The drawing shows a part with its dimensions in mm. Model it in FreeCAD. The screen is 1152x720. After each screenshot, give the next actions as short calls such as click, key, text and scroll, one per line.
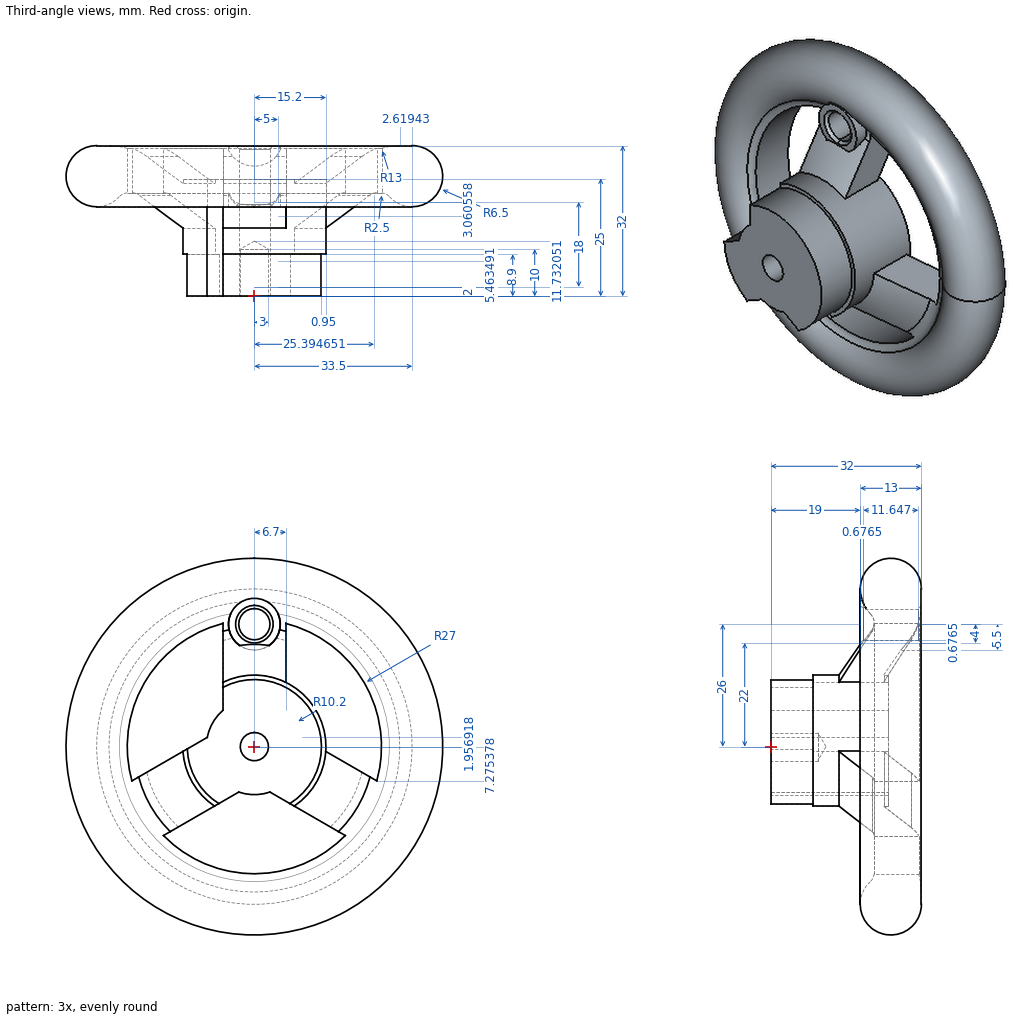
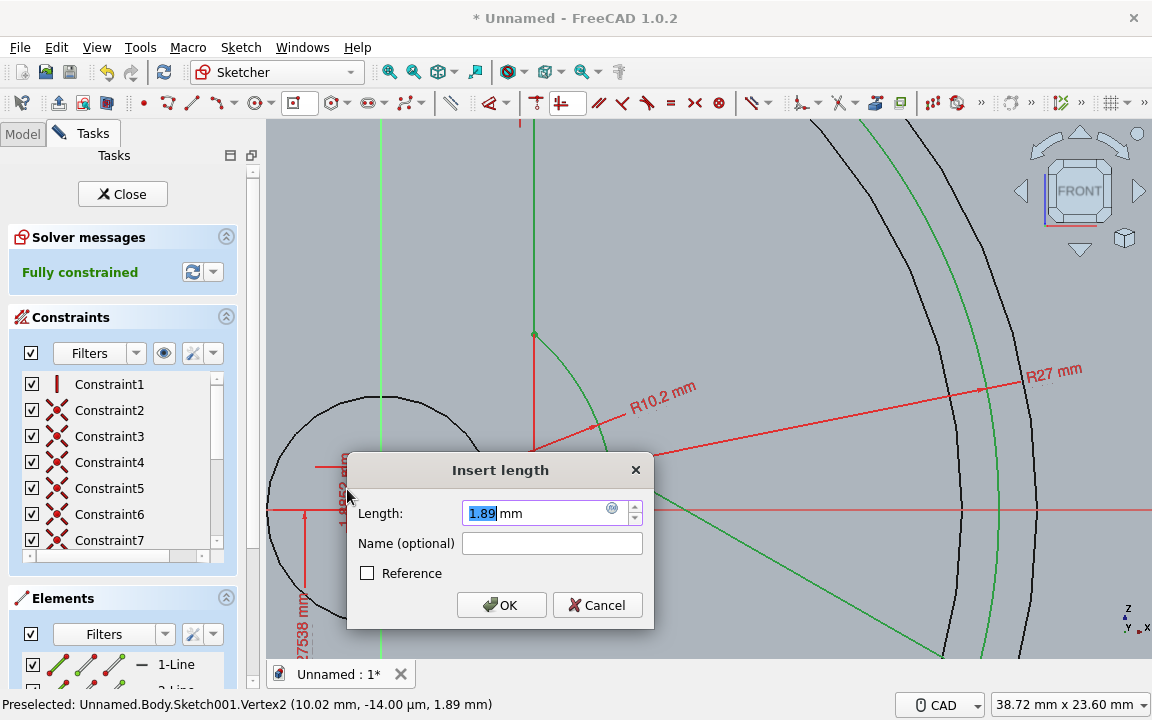
text(1.956918)
key(Return)
key(Escape)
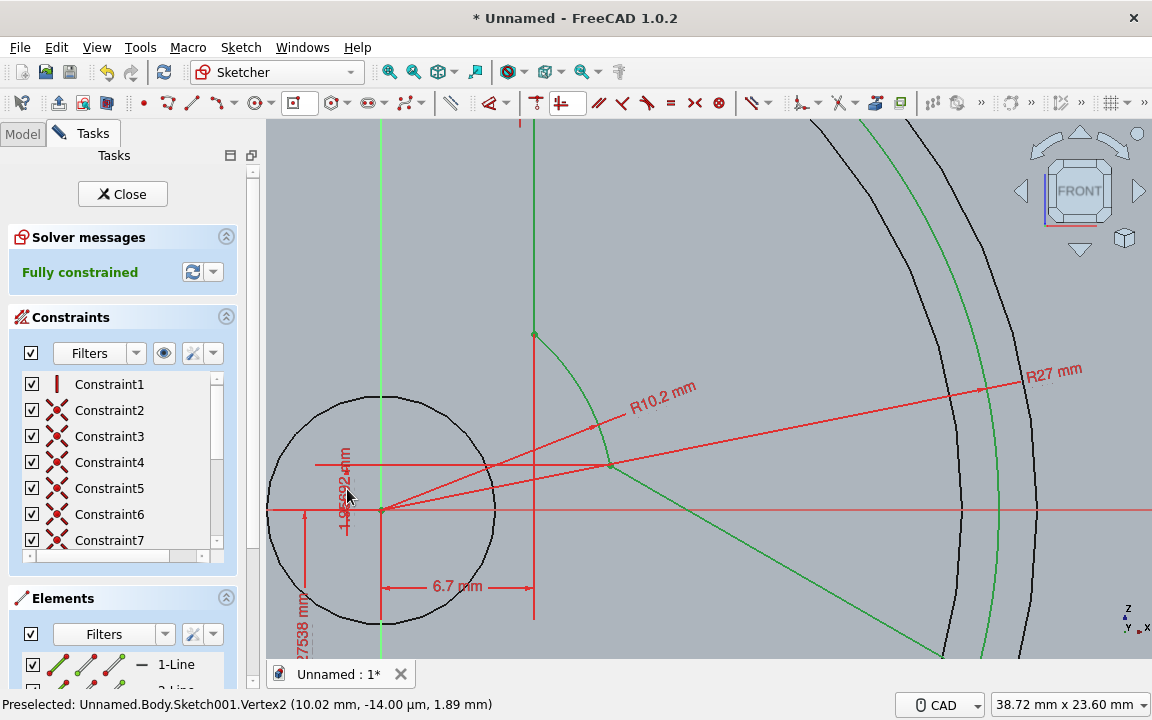
click(123, 194)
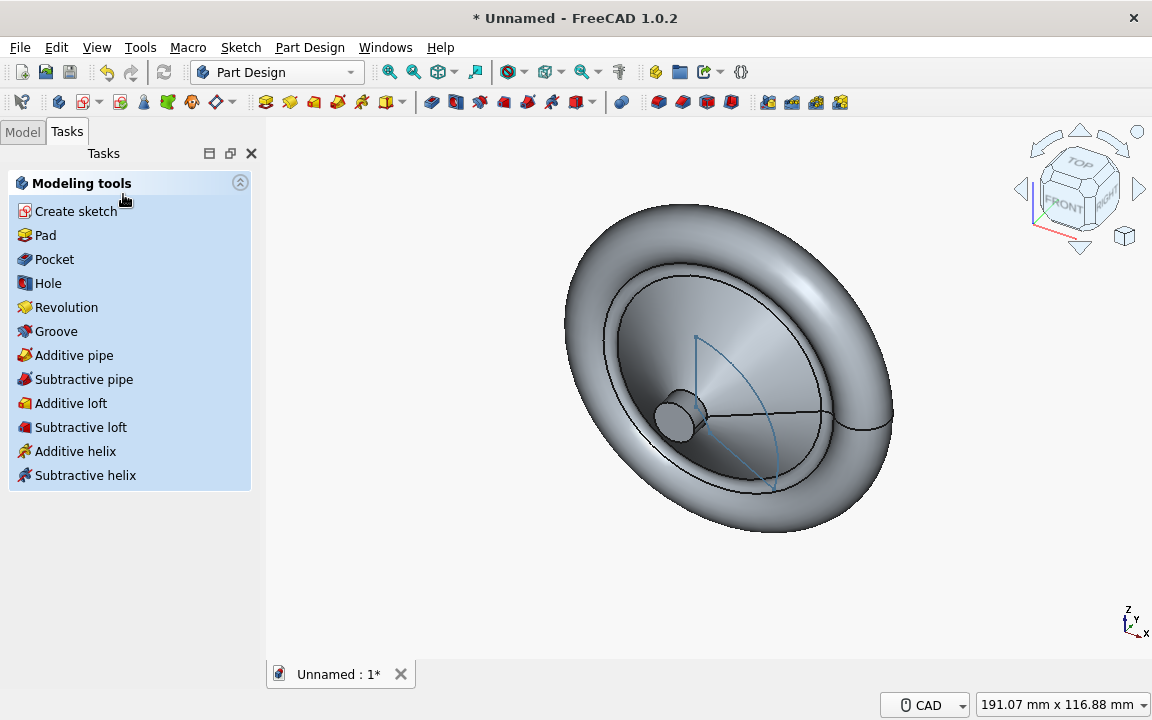
click(432, 102)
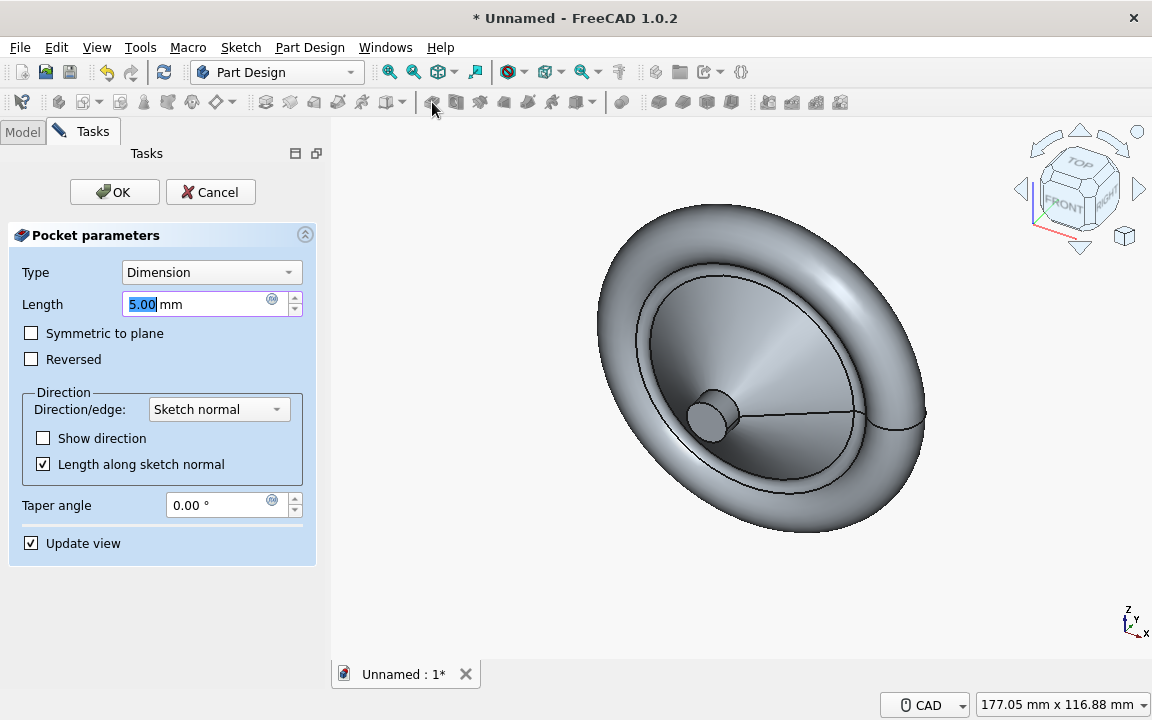
text(32)
key(Tab)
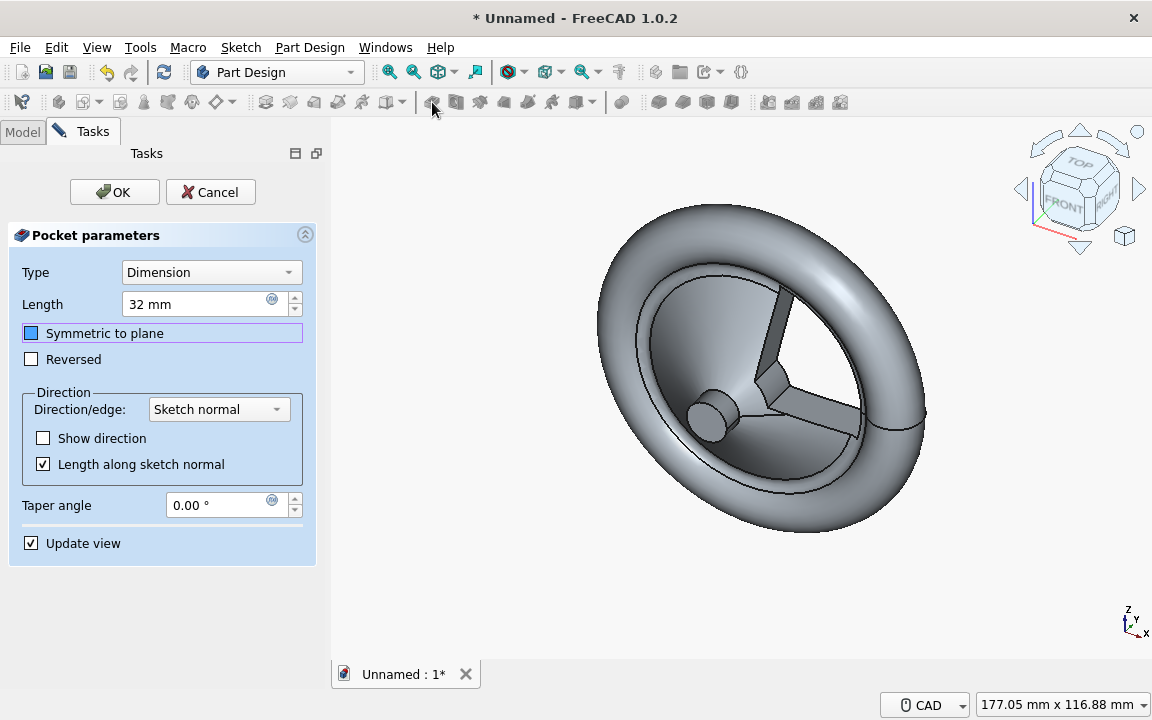
click(115, 192)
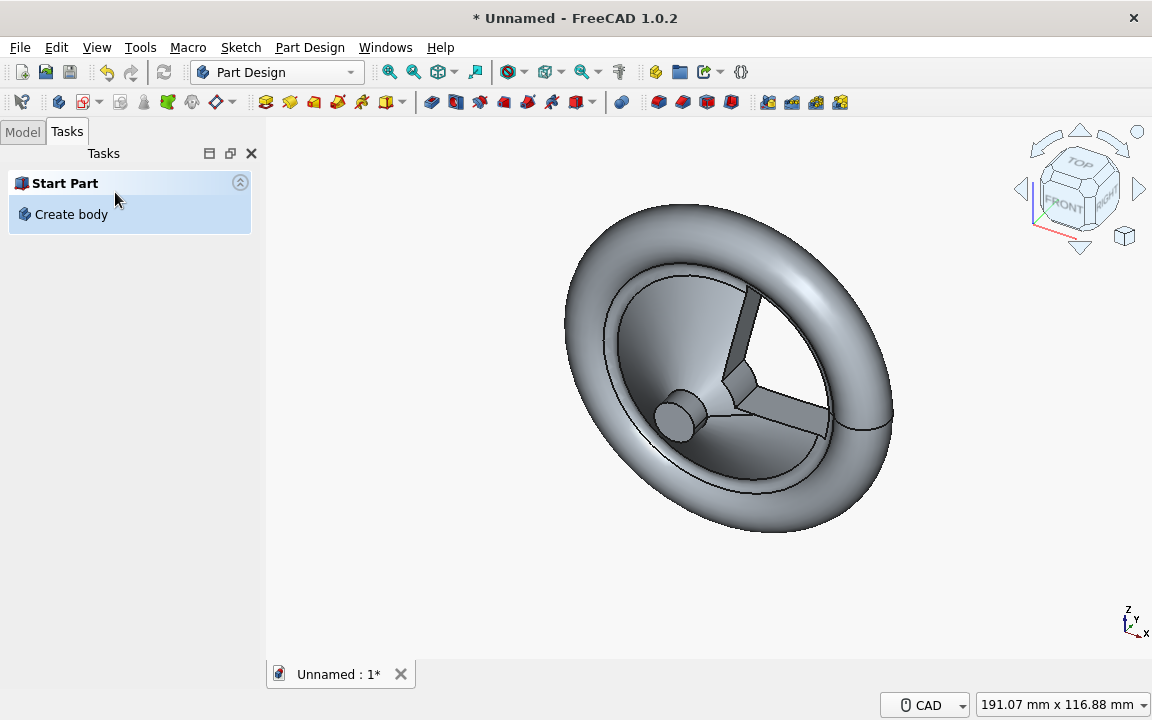
click(84, 102)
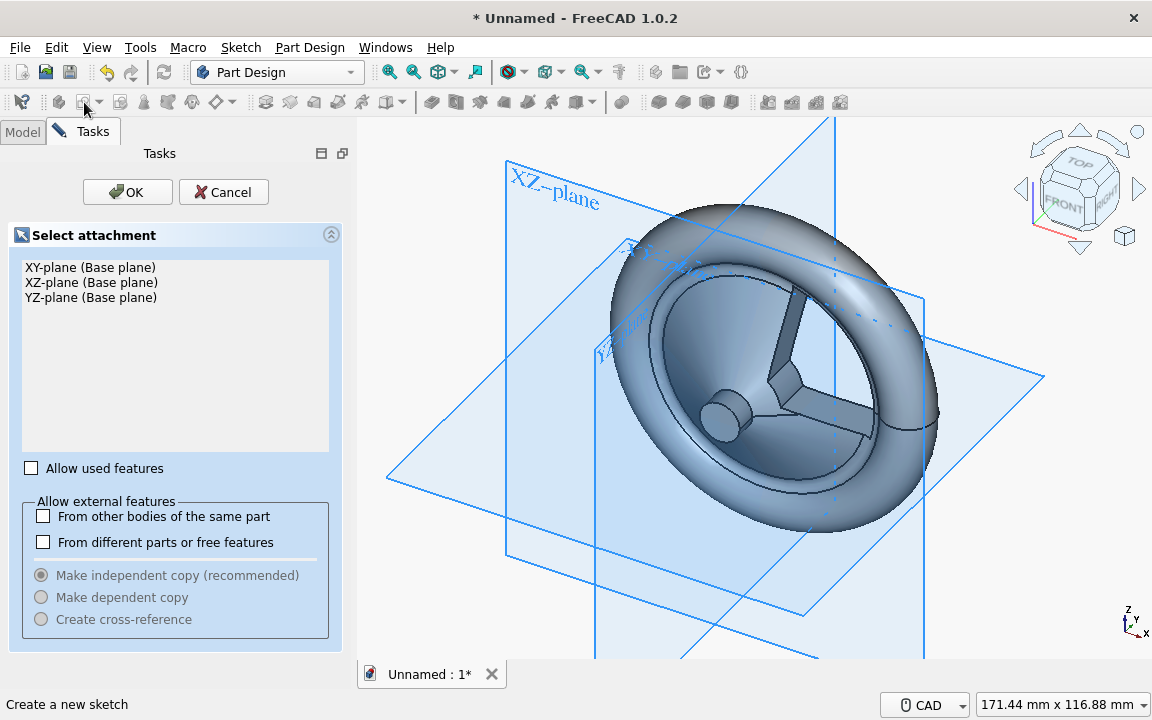
click(82, 268)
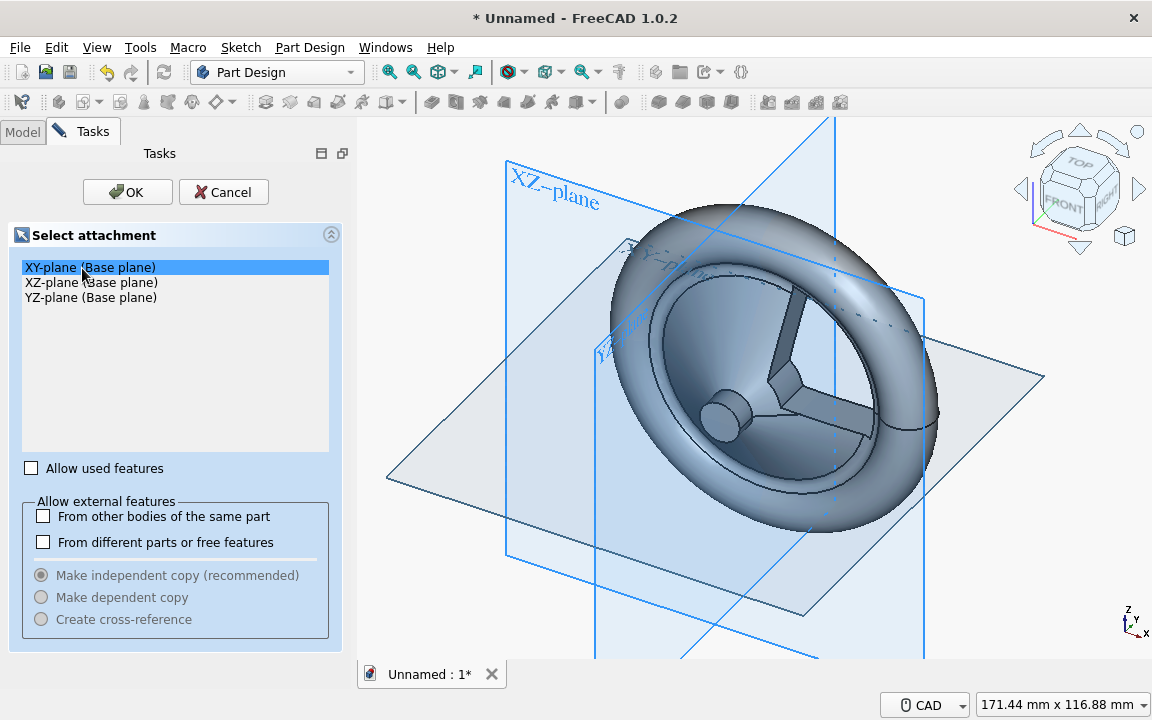
click(128, 192)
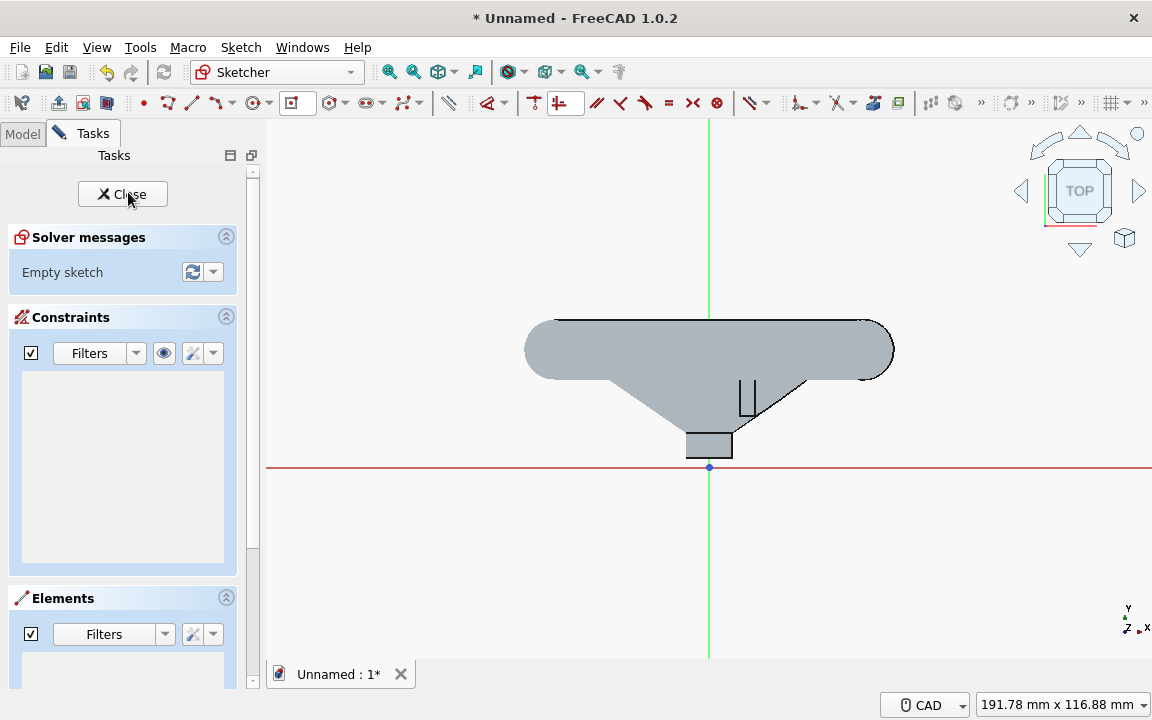
click(108, 104)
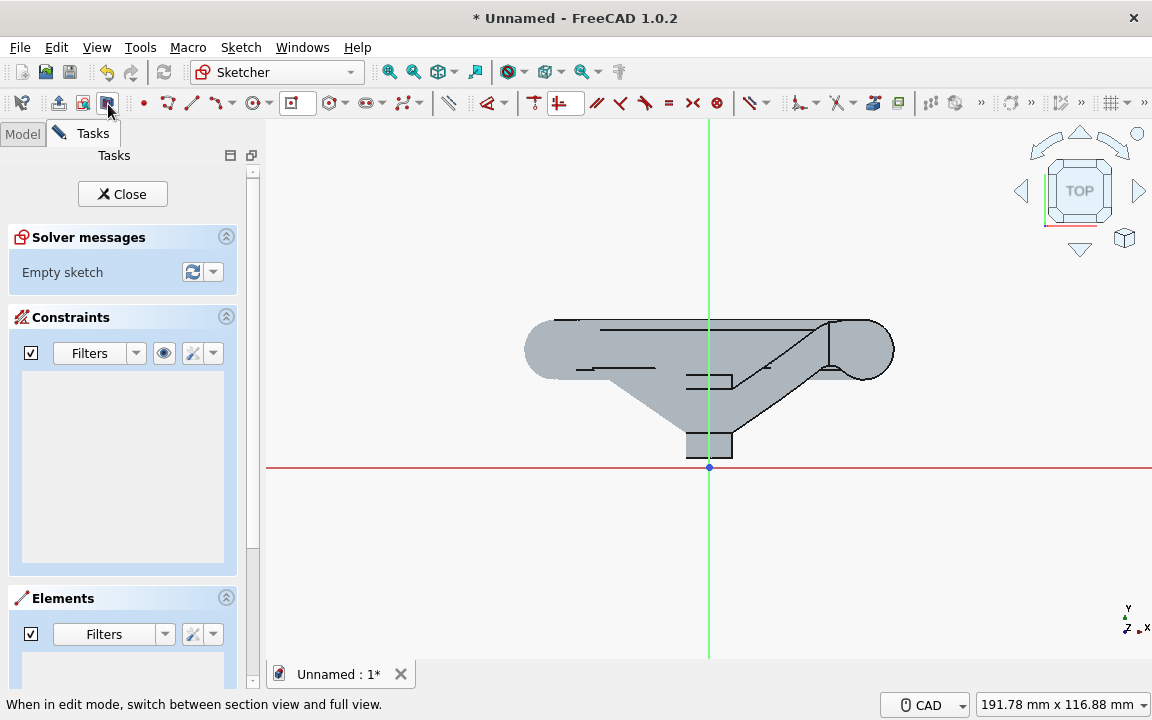
scroll(804, 422, up, 5)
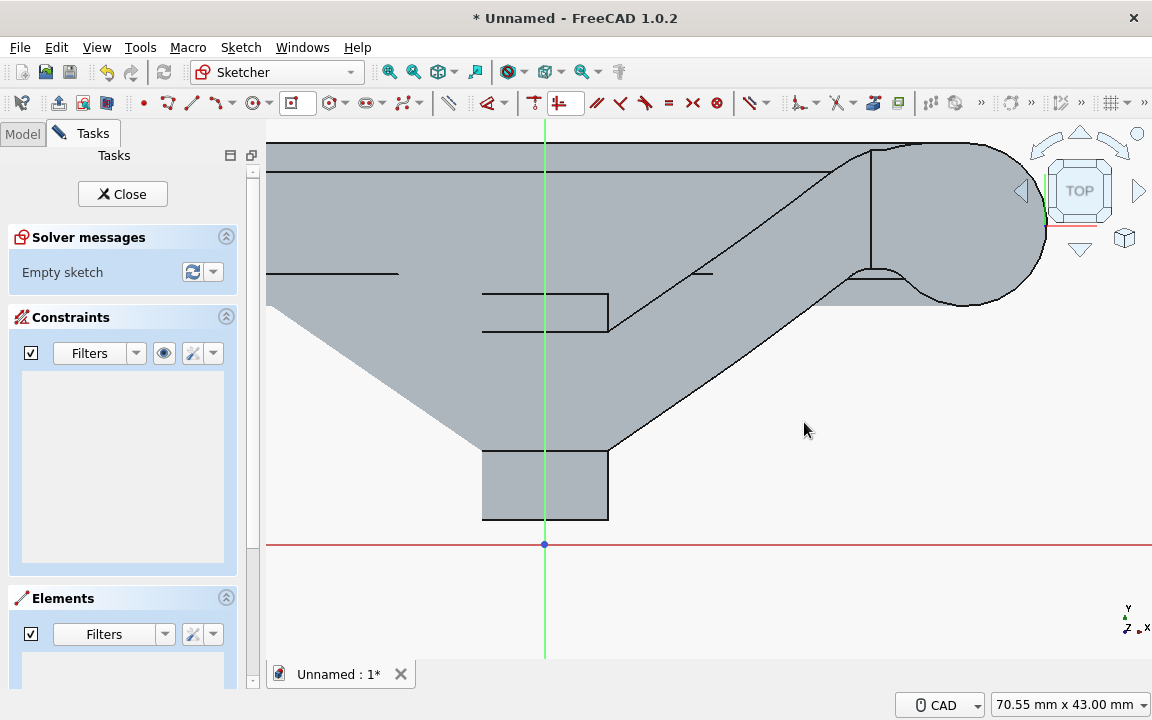
key(g)
key(m)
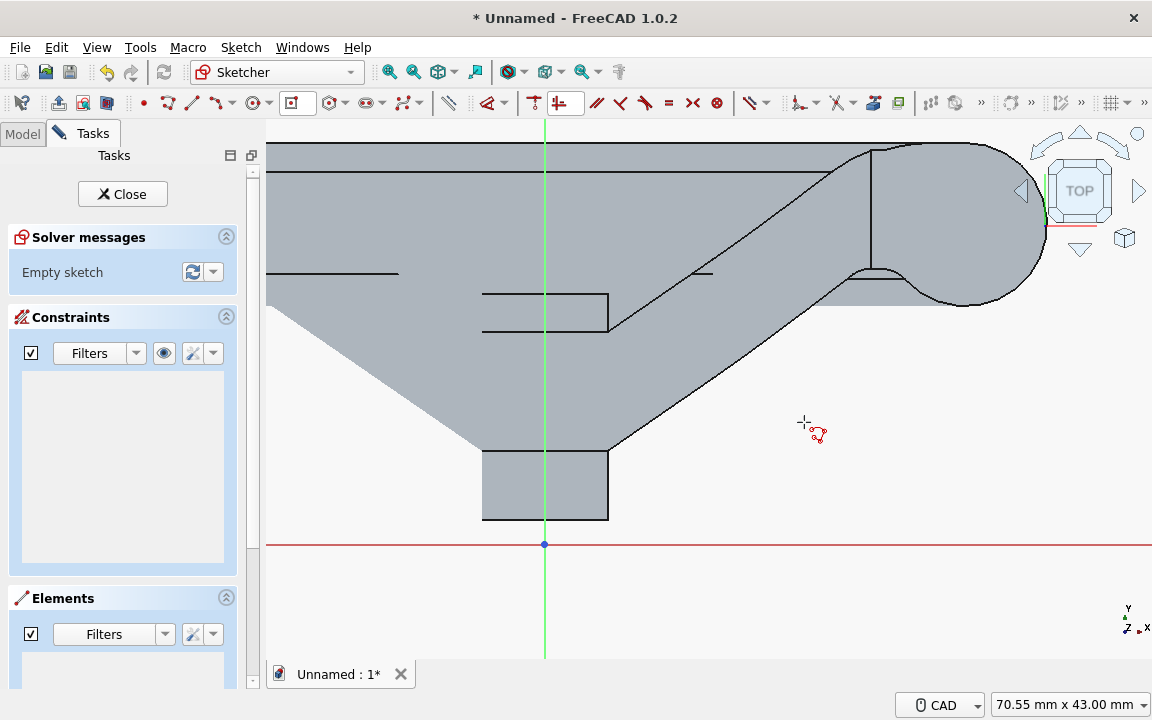
click(545, 545)
click(724, 536)
click(724, 433)